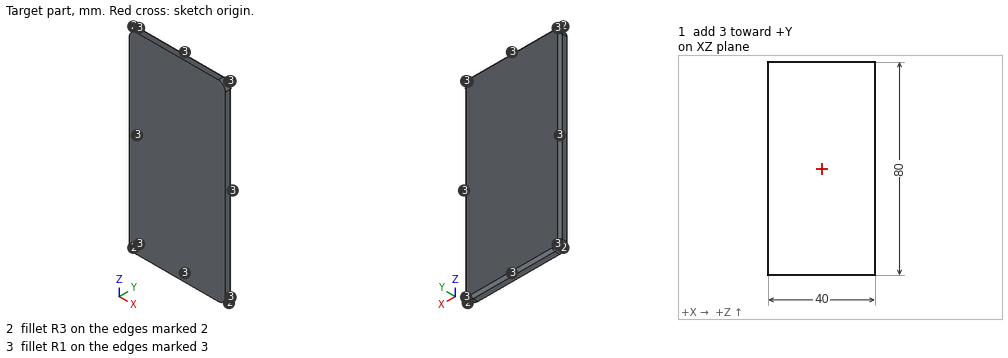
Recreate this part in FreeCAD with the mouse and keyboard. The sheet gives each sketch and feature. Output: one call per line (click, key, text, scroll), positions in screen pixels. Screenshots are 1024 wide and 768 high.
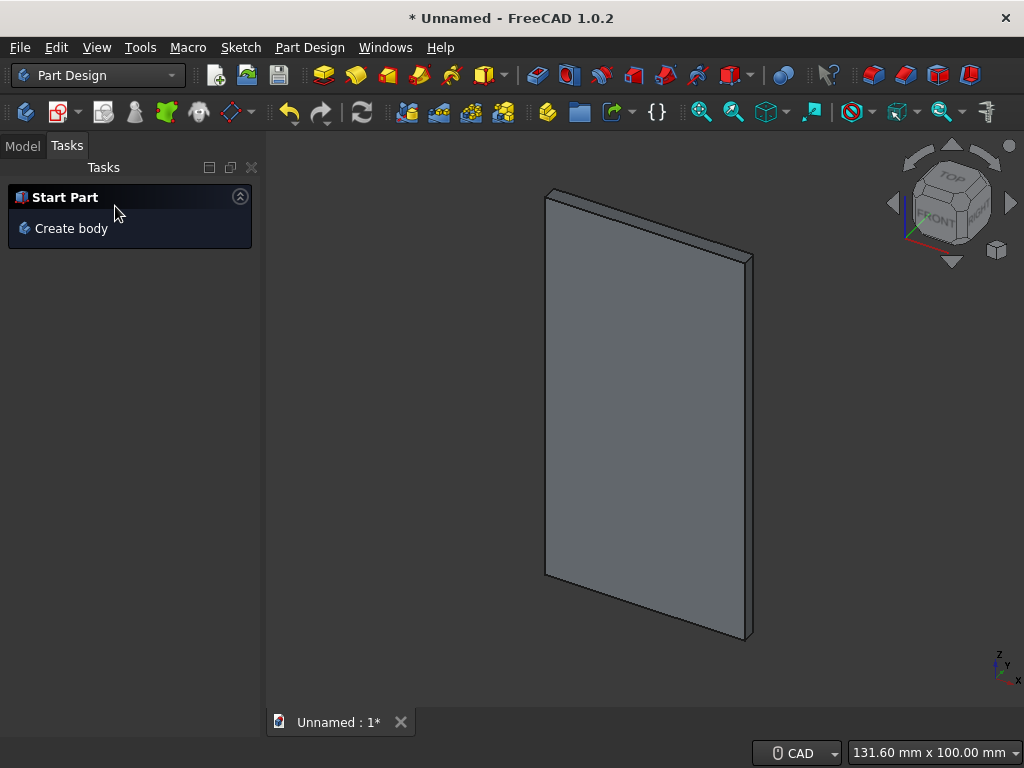
click(750, 257)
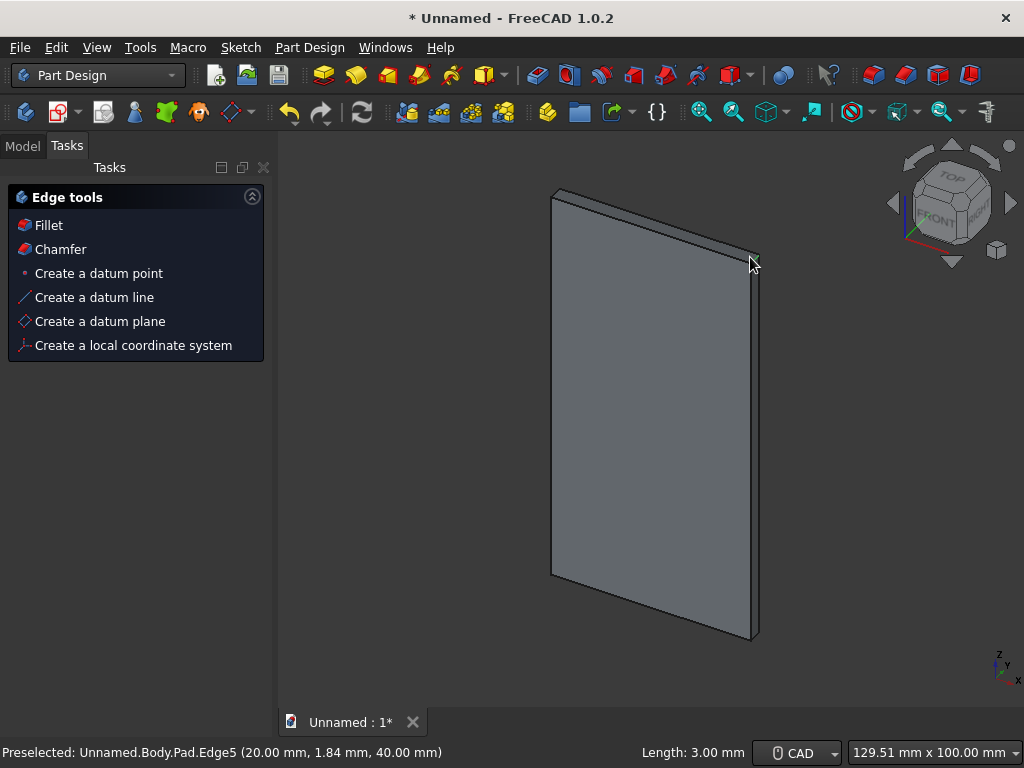
scroll(556, 192, up, 5)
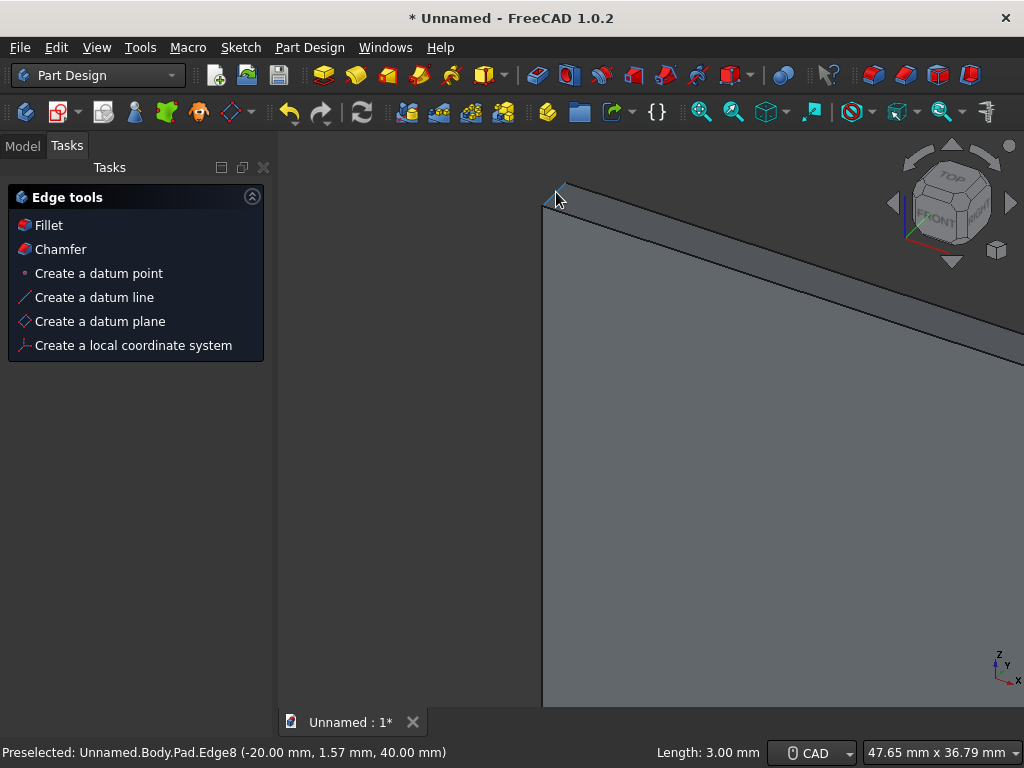
key(v)
key(f)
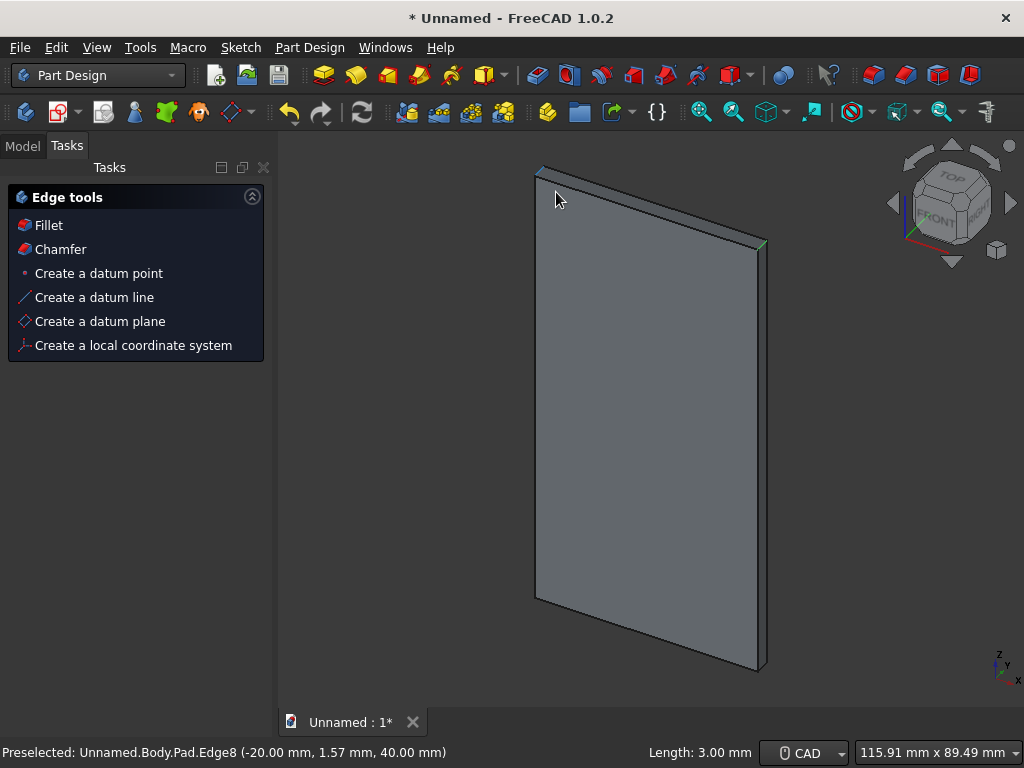
key(0)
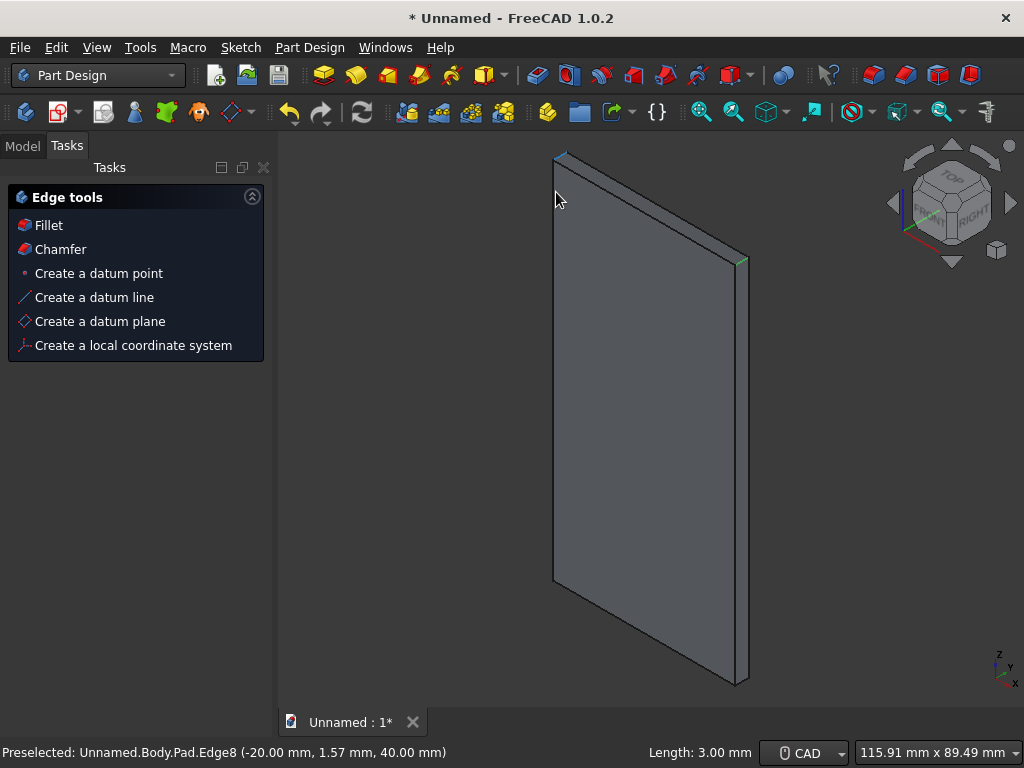
key(2)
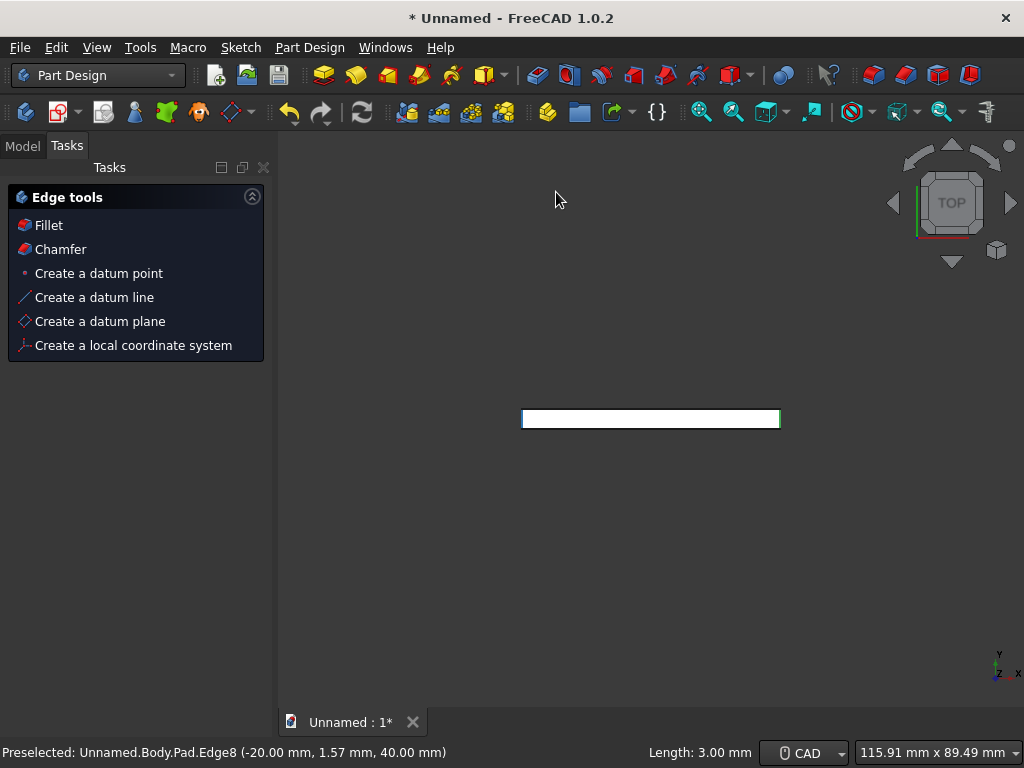
key(v)
key(f)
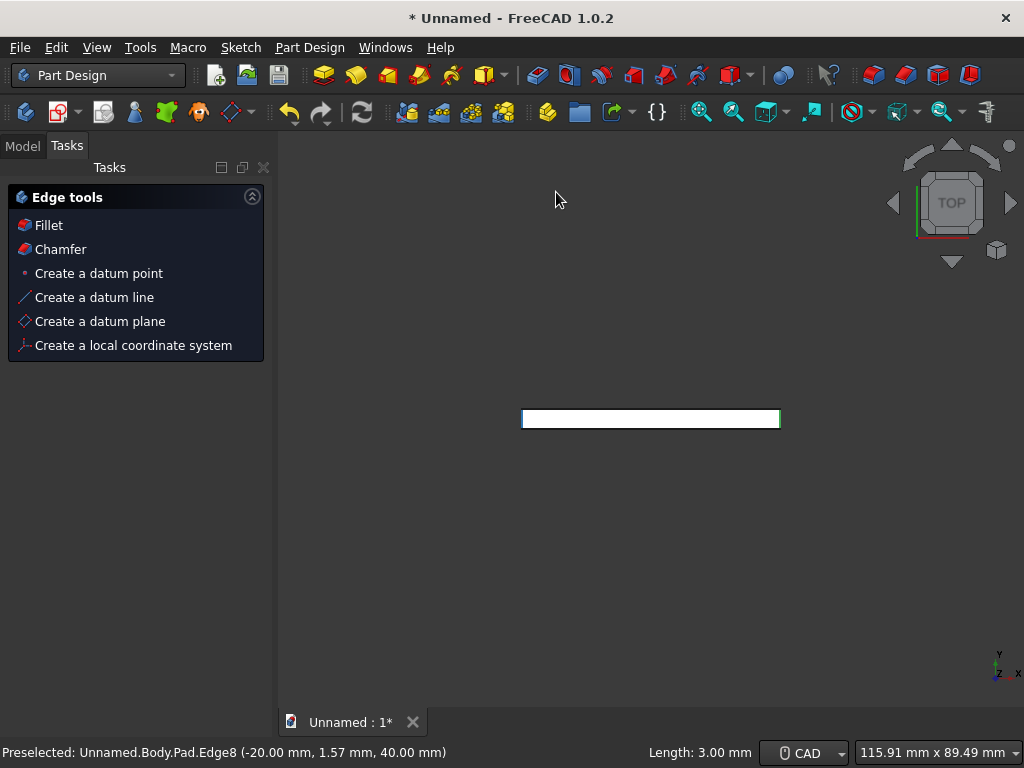
click(522, 418, ctrl)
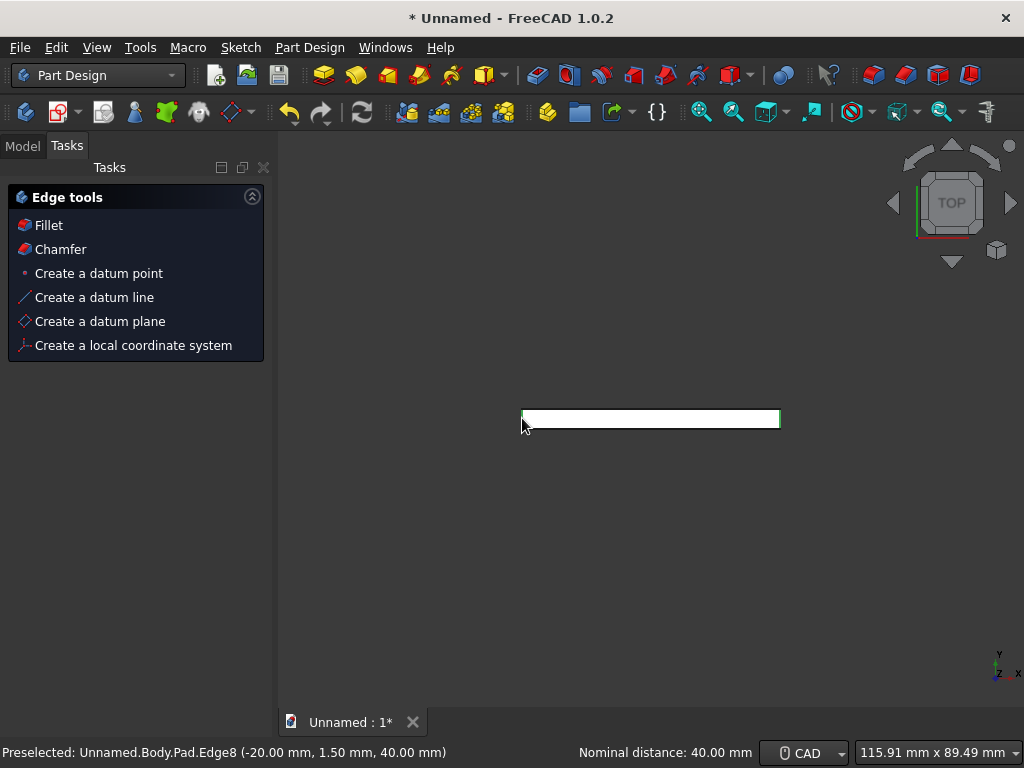
scroll(522, 418, up, 4)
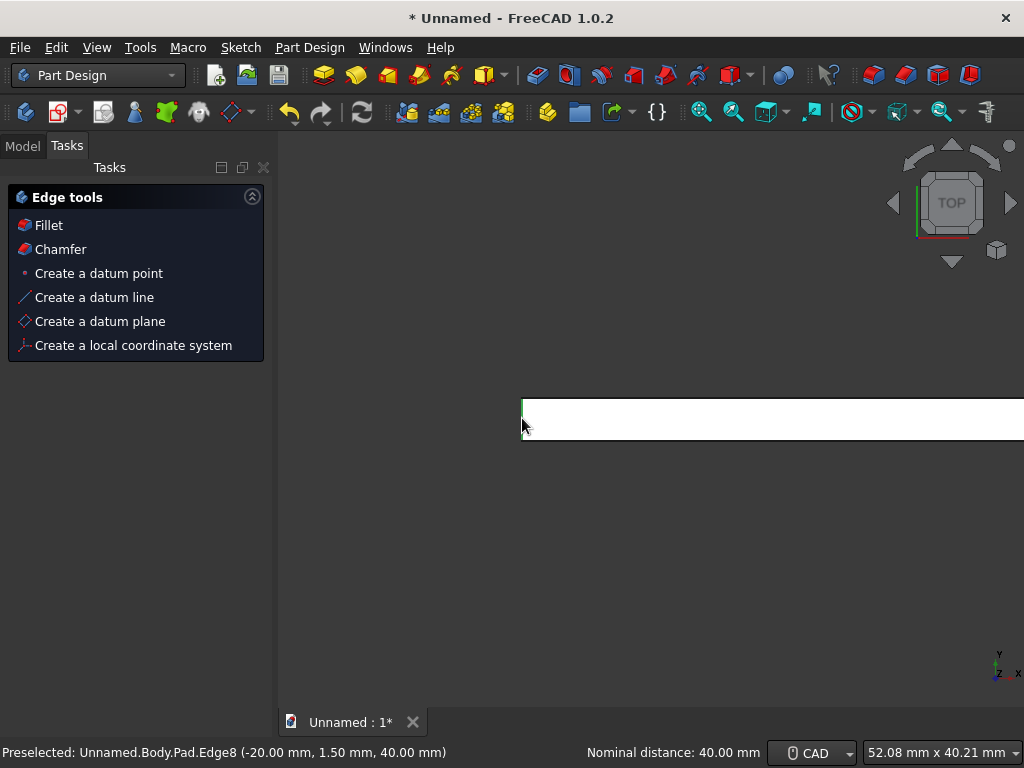
click(702, 112)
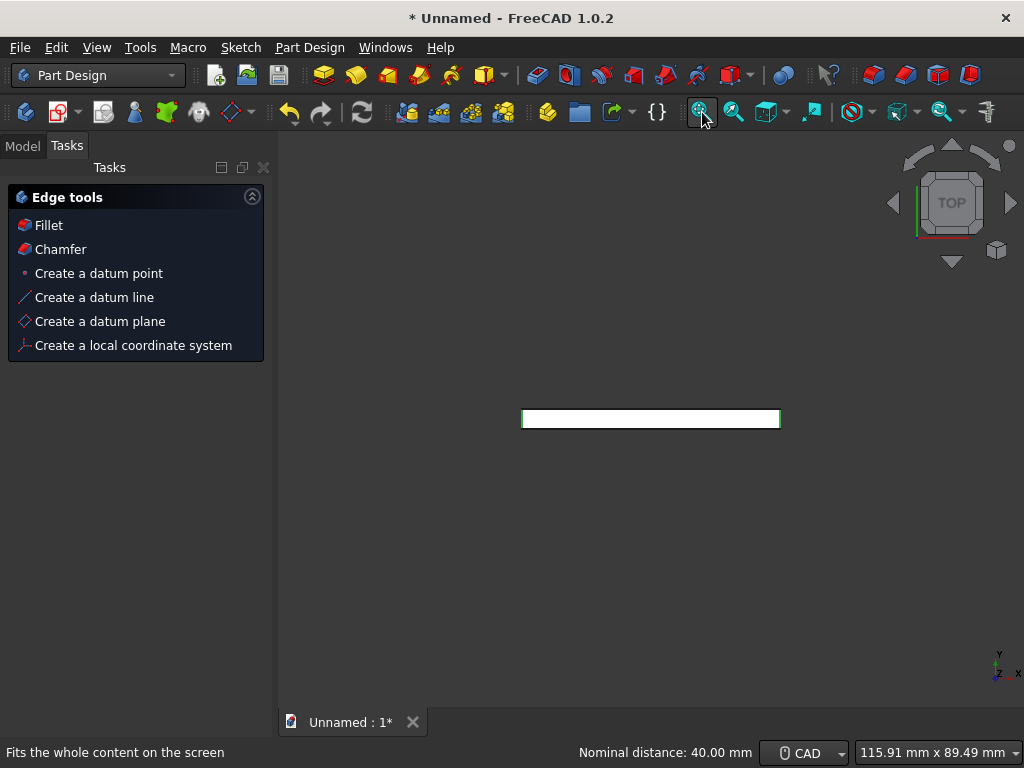
key(1)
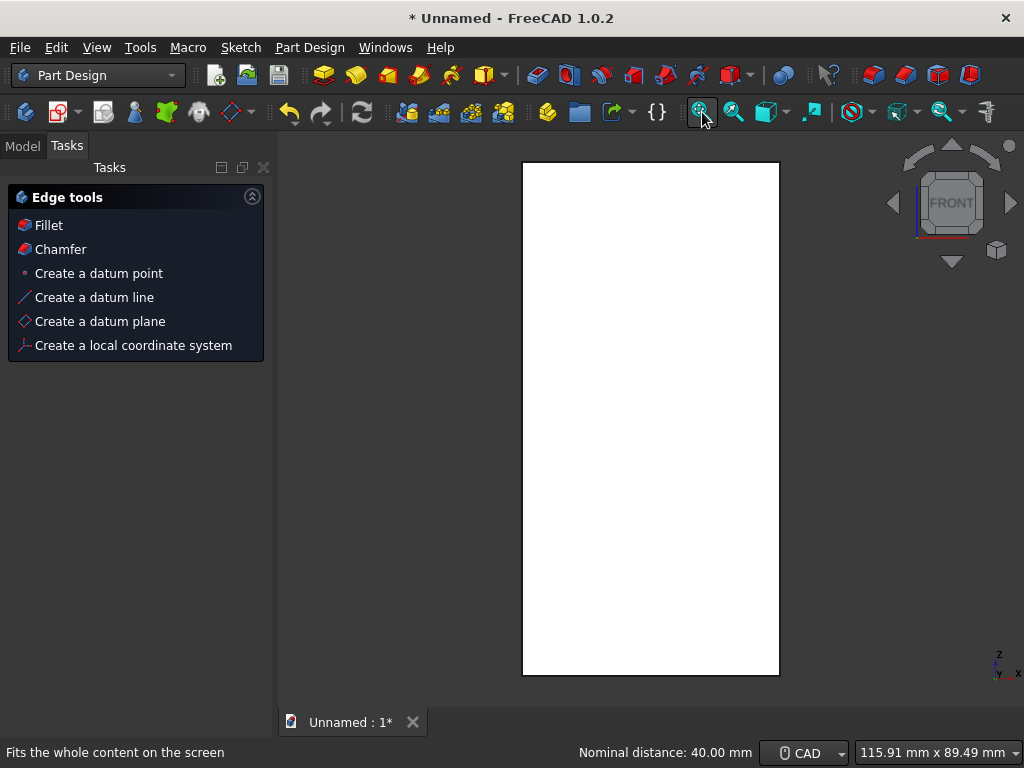
scroll(522, 675, up, 4)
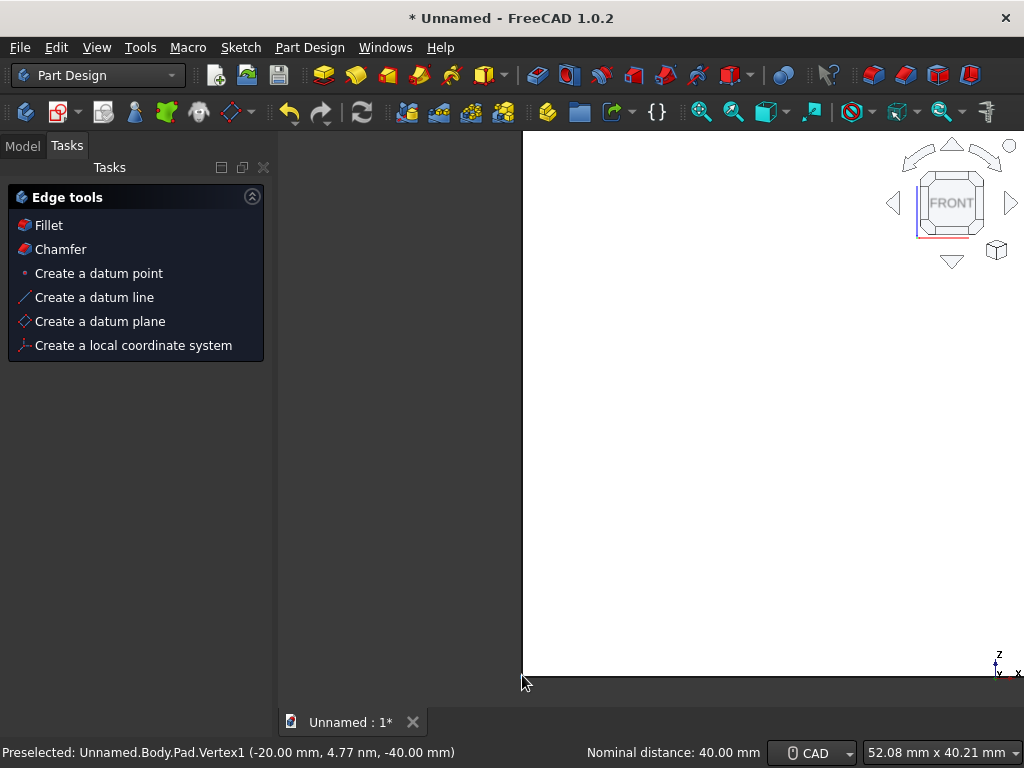
key(v)
key(f)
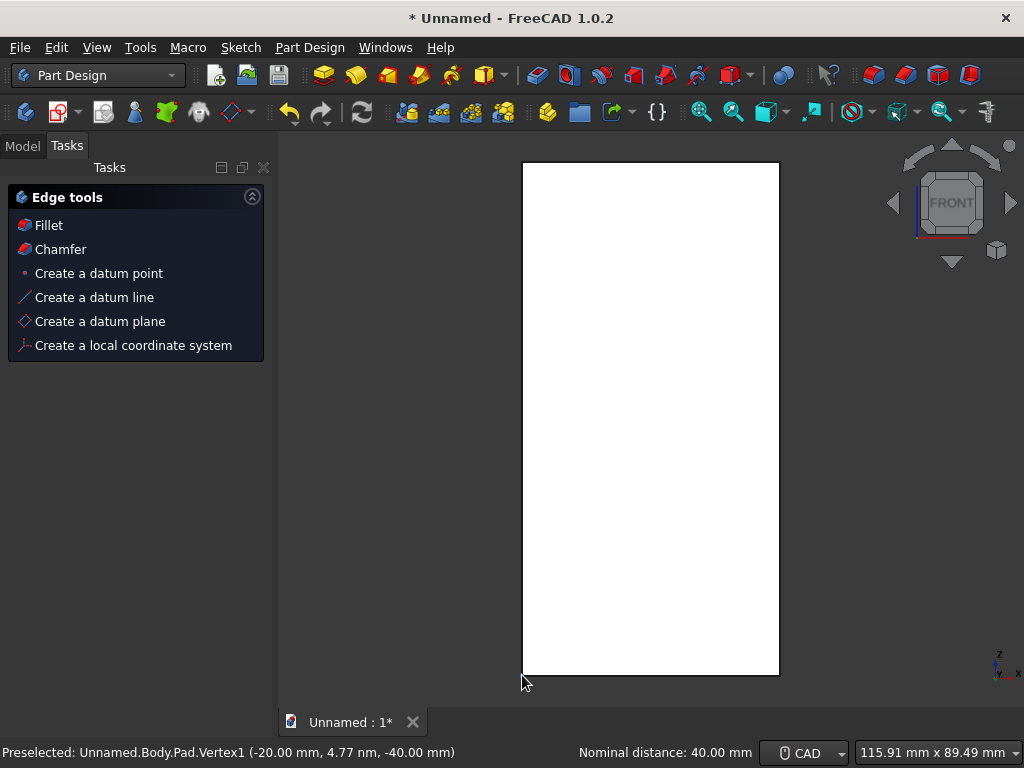
key(3)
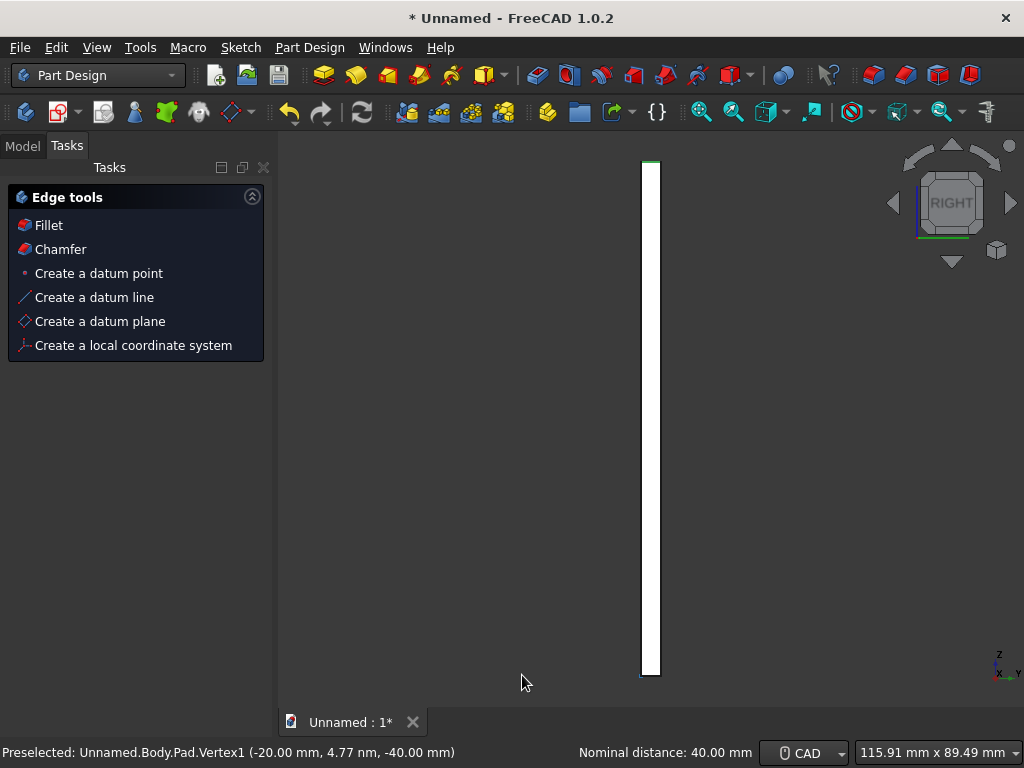
click(651, 675, ctrl)